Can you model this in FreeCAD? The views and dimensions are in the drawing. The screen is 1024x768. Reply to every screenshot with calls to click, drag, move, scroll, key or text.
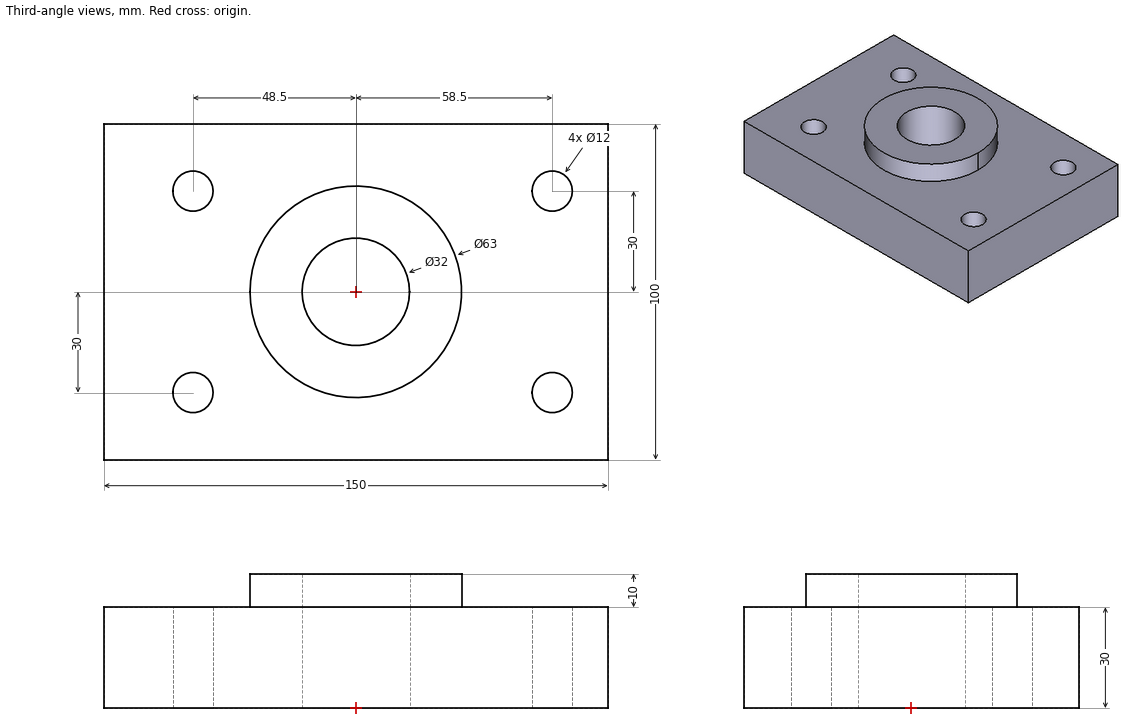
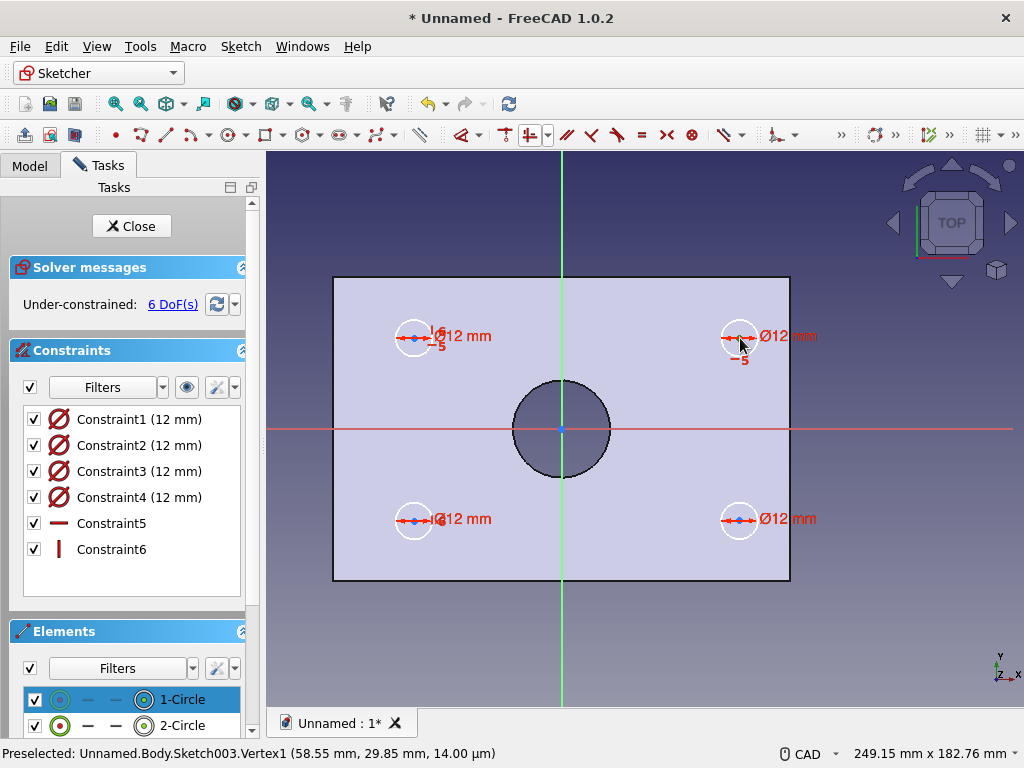
click(740, 521)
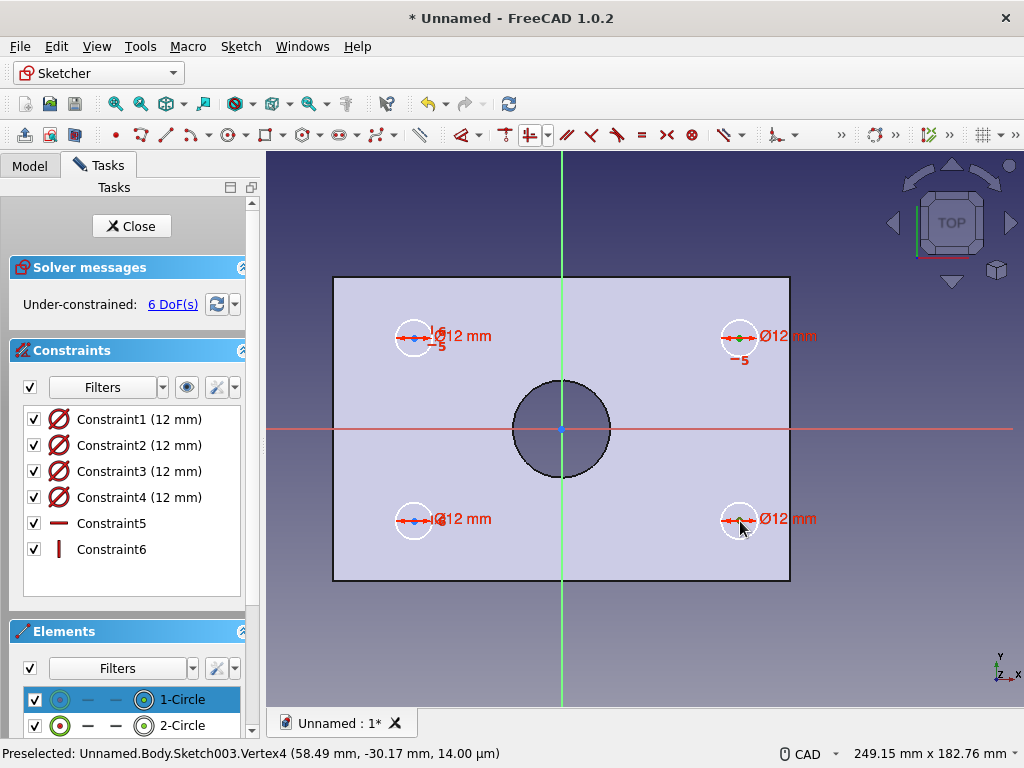
click(548, 136)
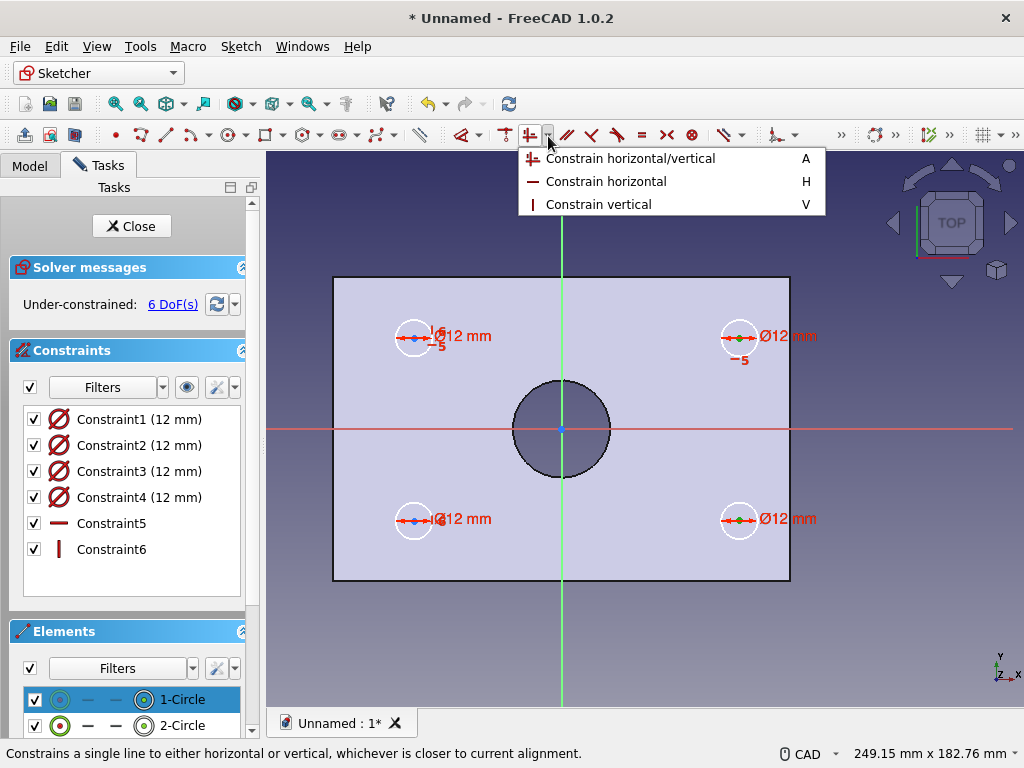
click(672, 204)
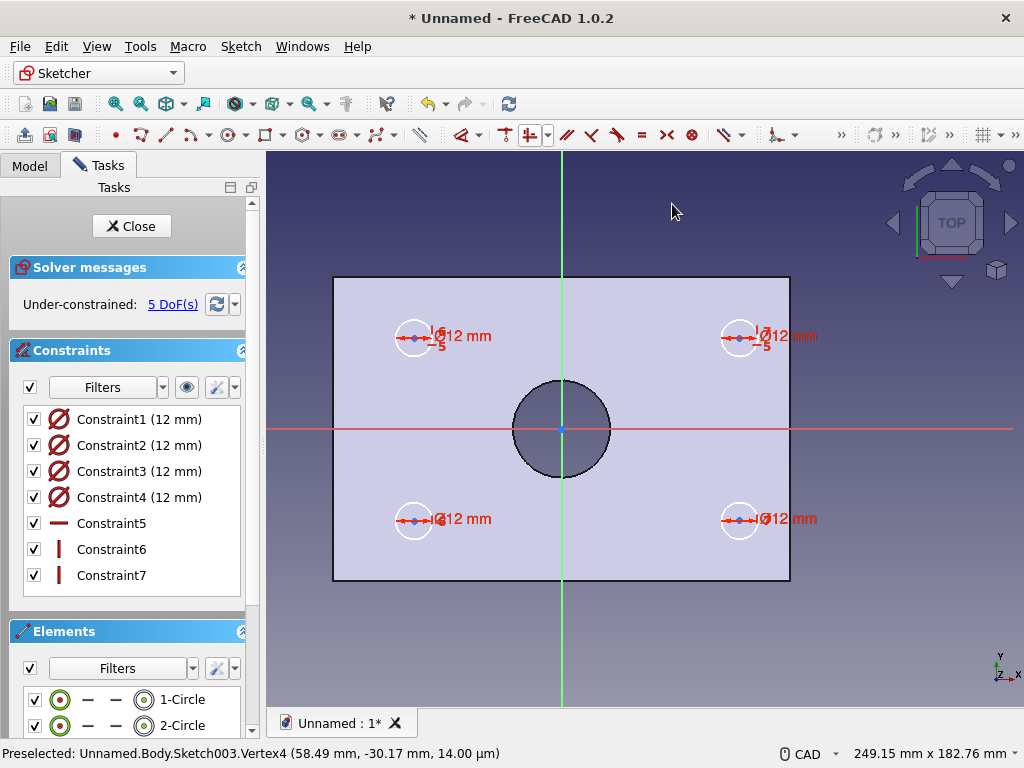
click(414, 521)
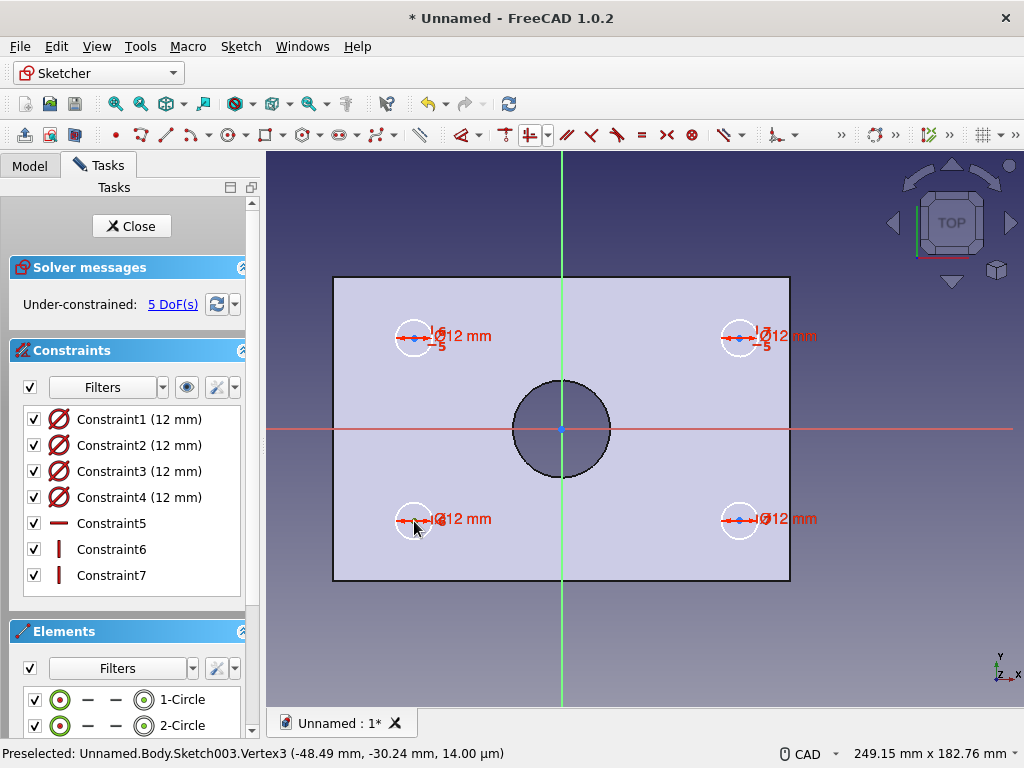
click(740, 521)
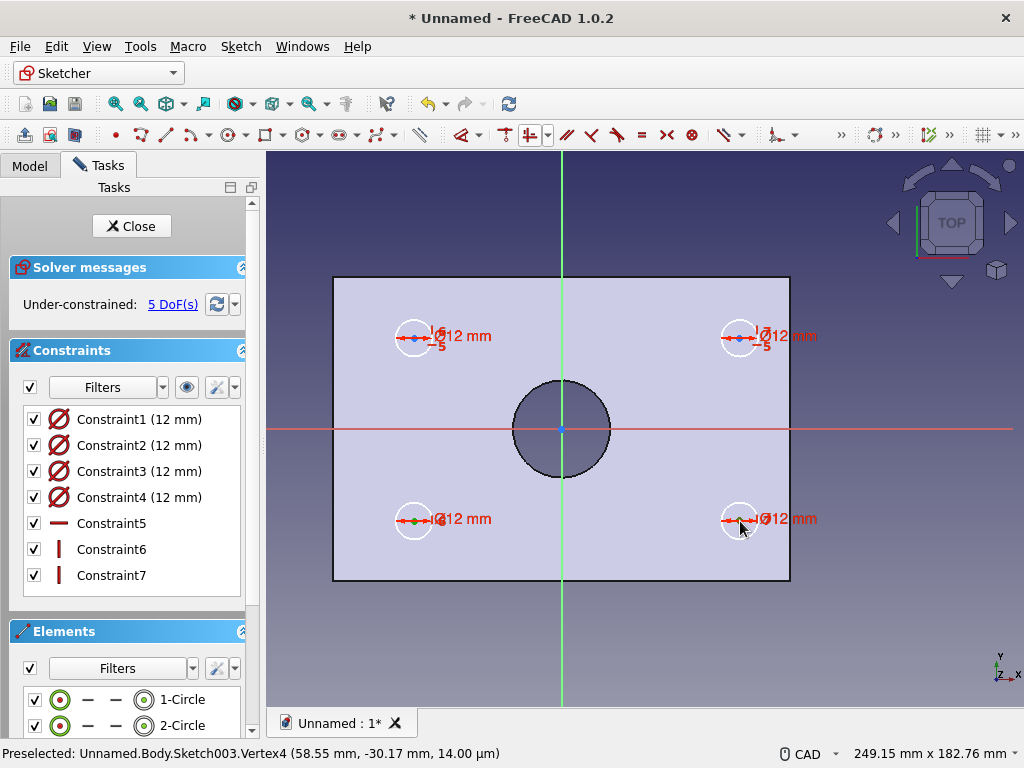
key(h)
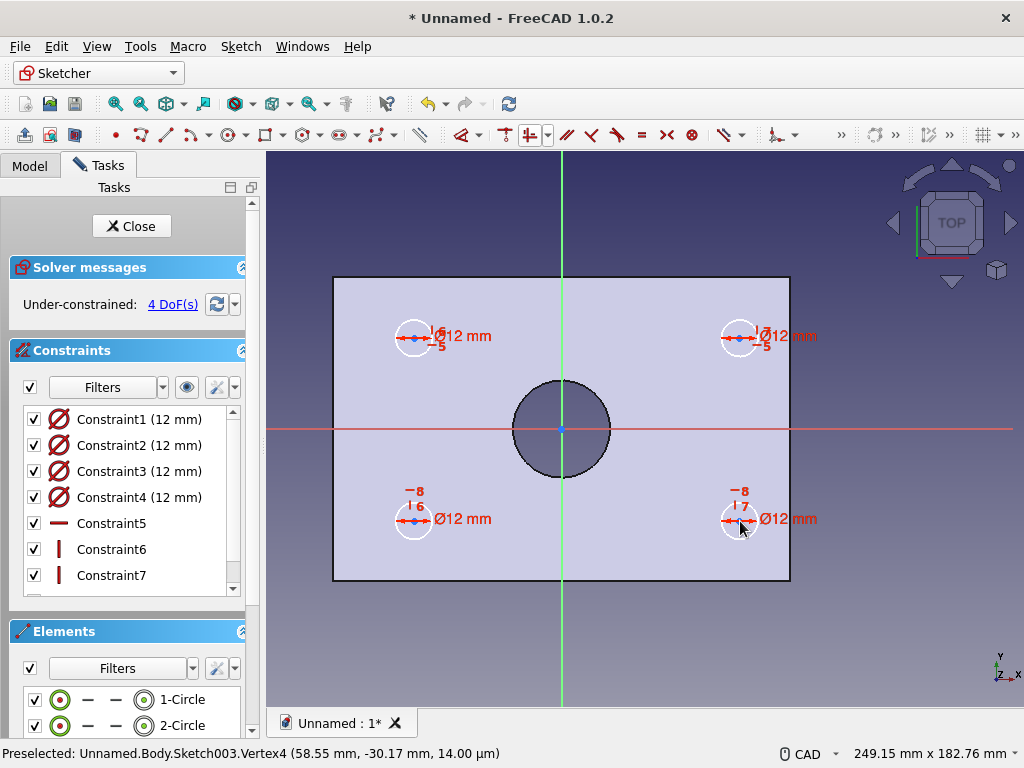
click(460, 136)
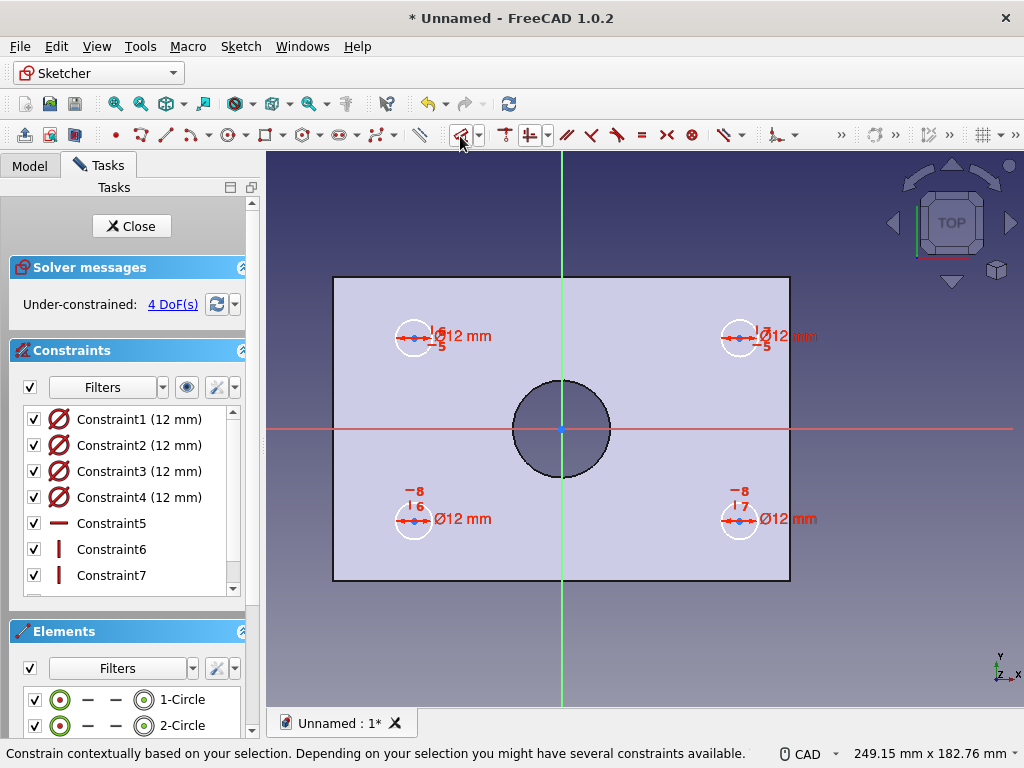
click(740, 338)
click(774, 384)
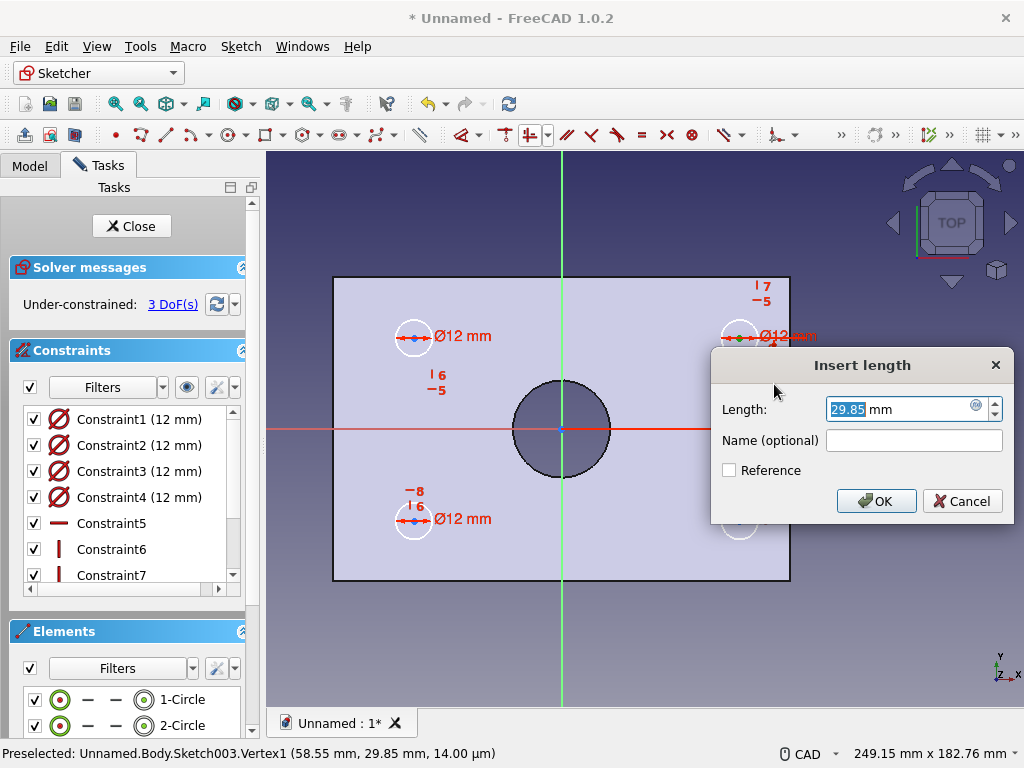
text(30)
key(Return)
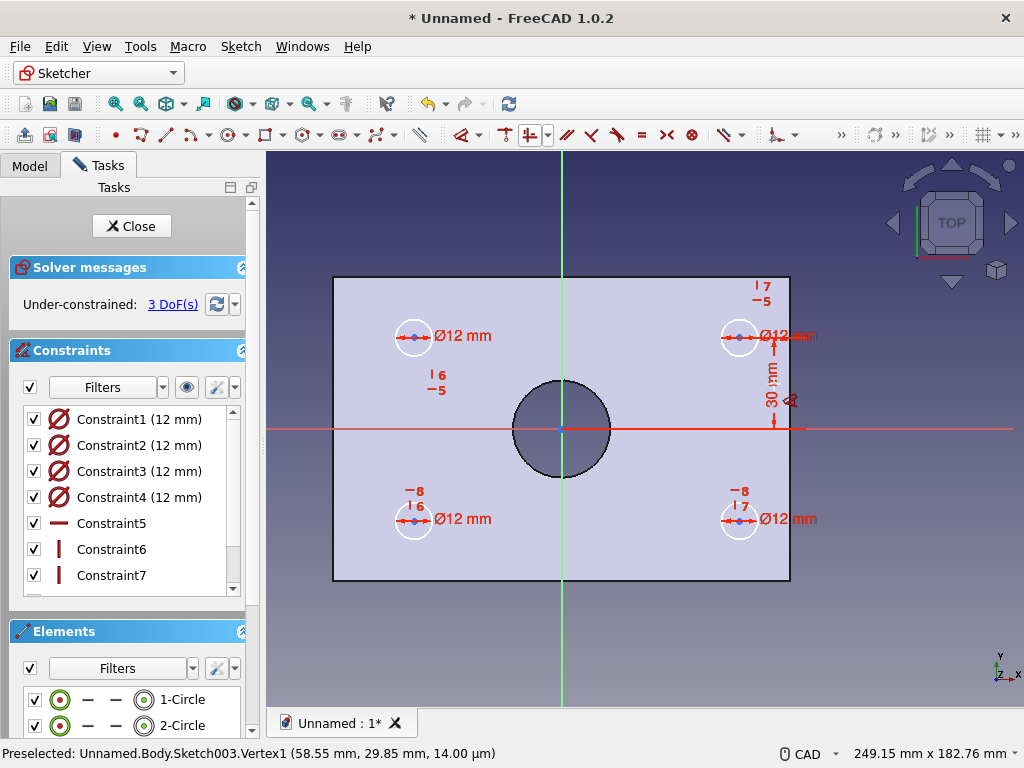
click(414, 521)
click(380, 475)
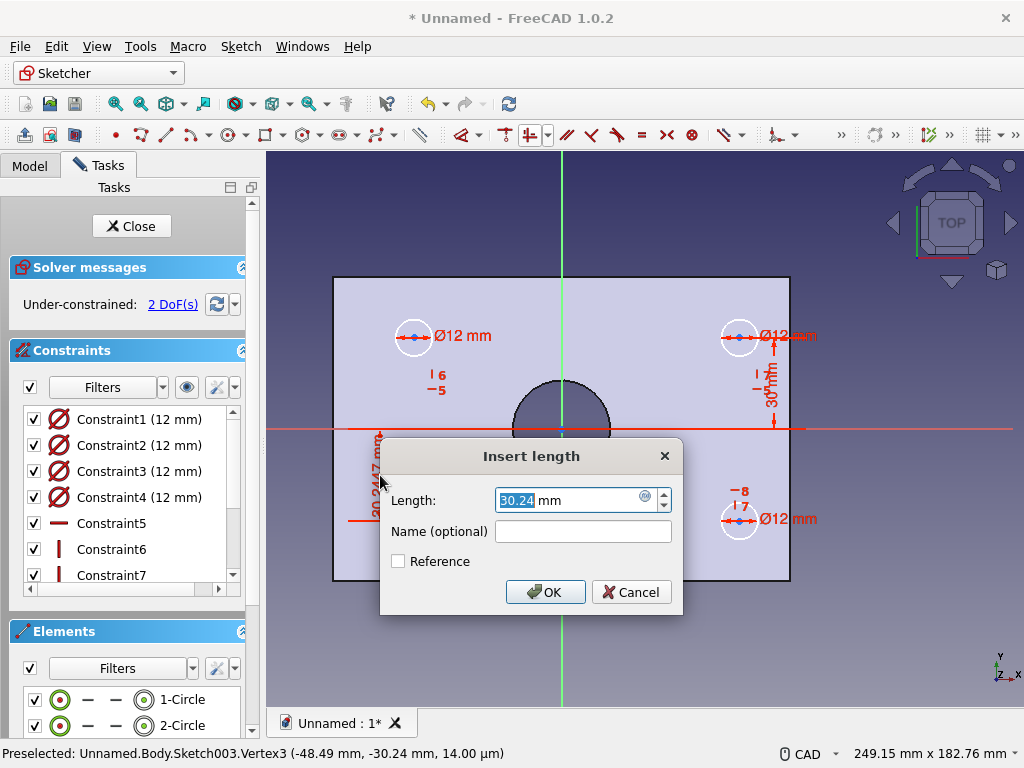
text(30)
key(Return)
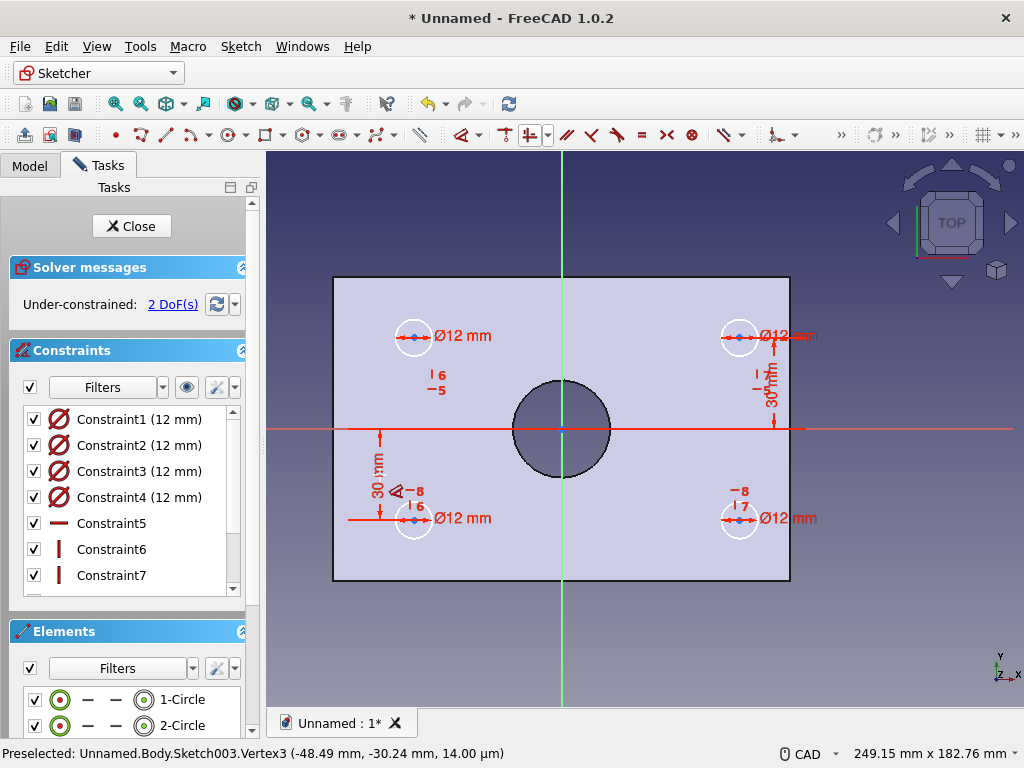
click(740, 338)
click(651, 304)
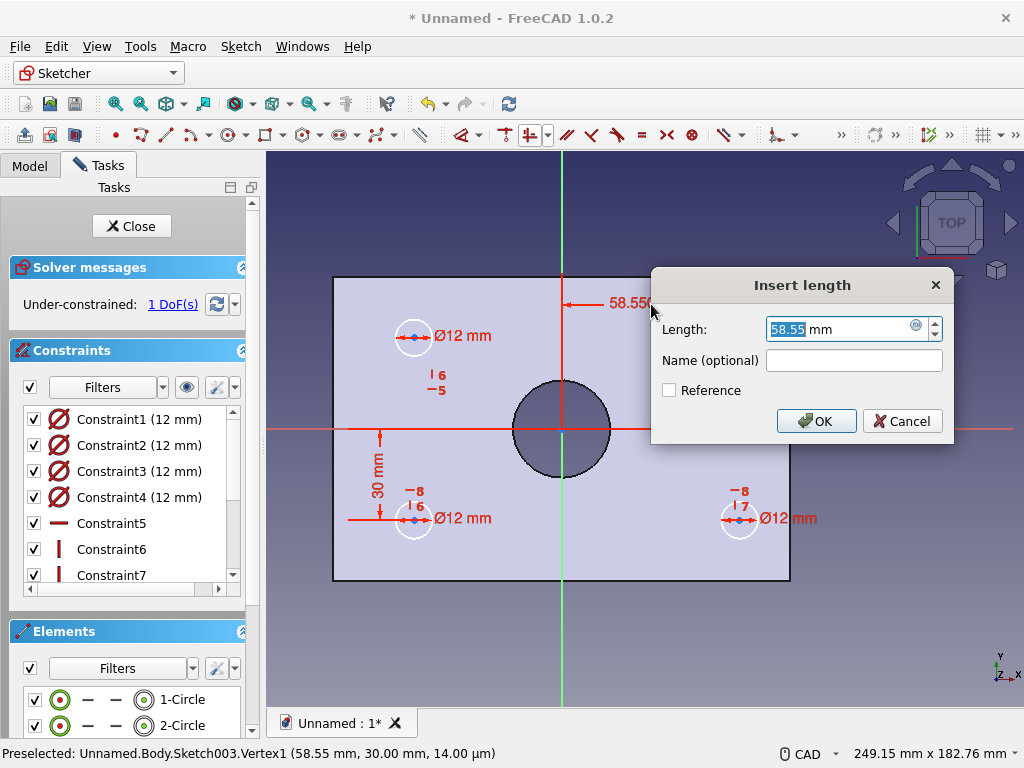
text(58.5)
key(Return)